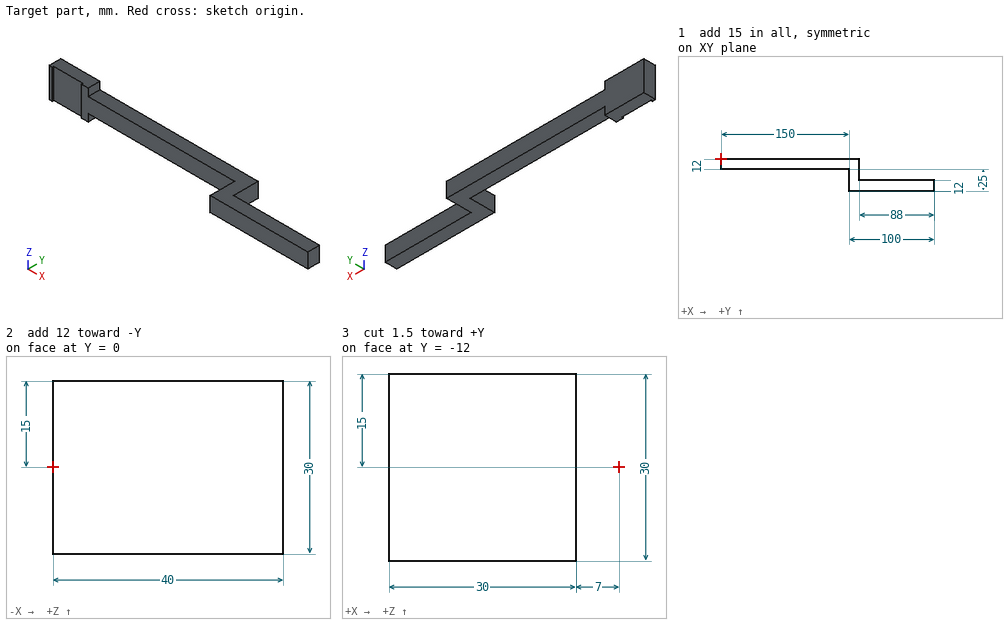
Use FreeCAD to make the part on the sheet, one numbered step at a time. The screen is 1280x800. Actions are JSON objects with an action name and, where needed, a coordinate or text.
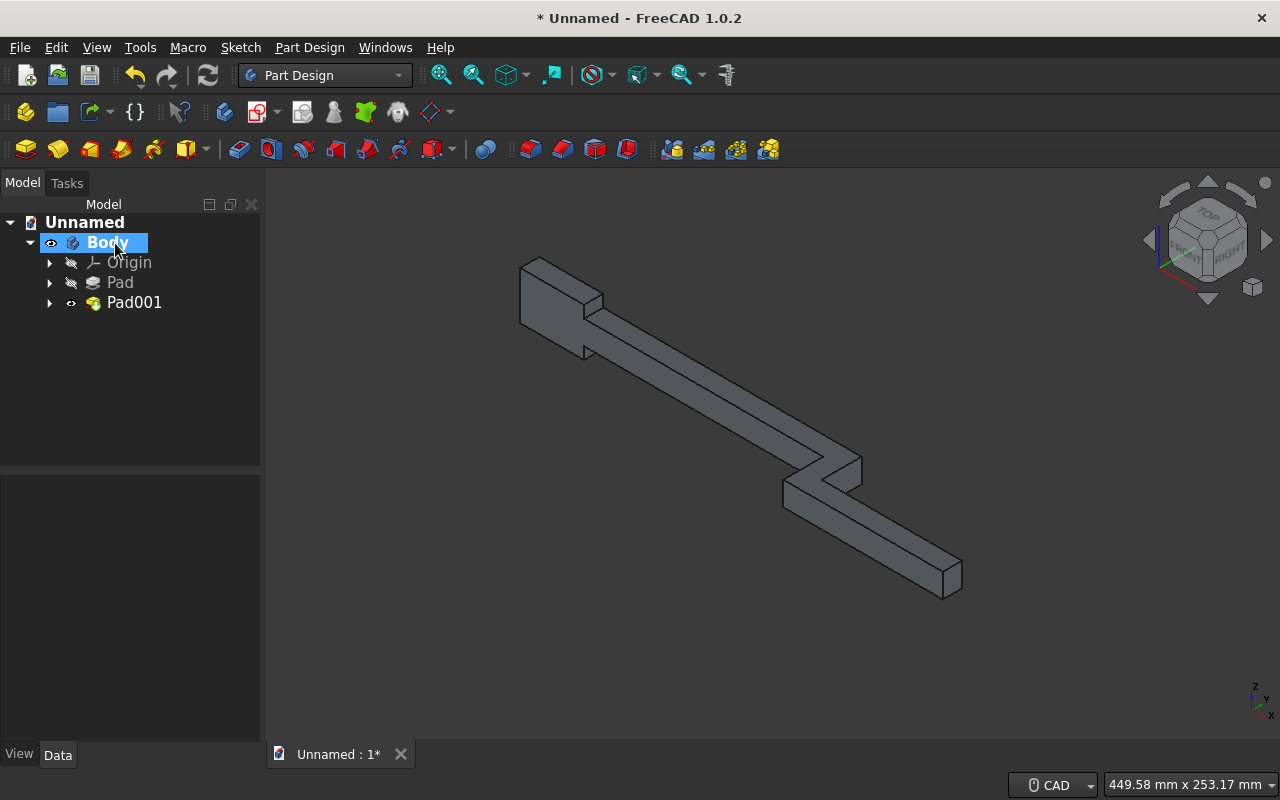
{"action": "left_click", "coordinate": [542, 307]}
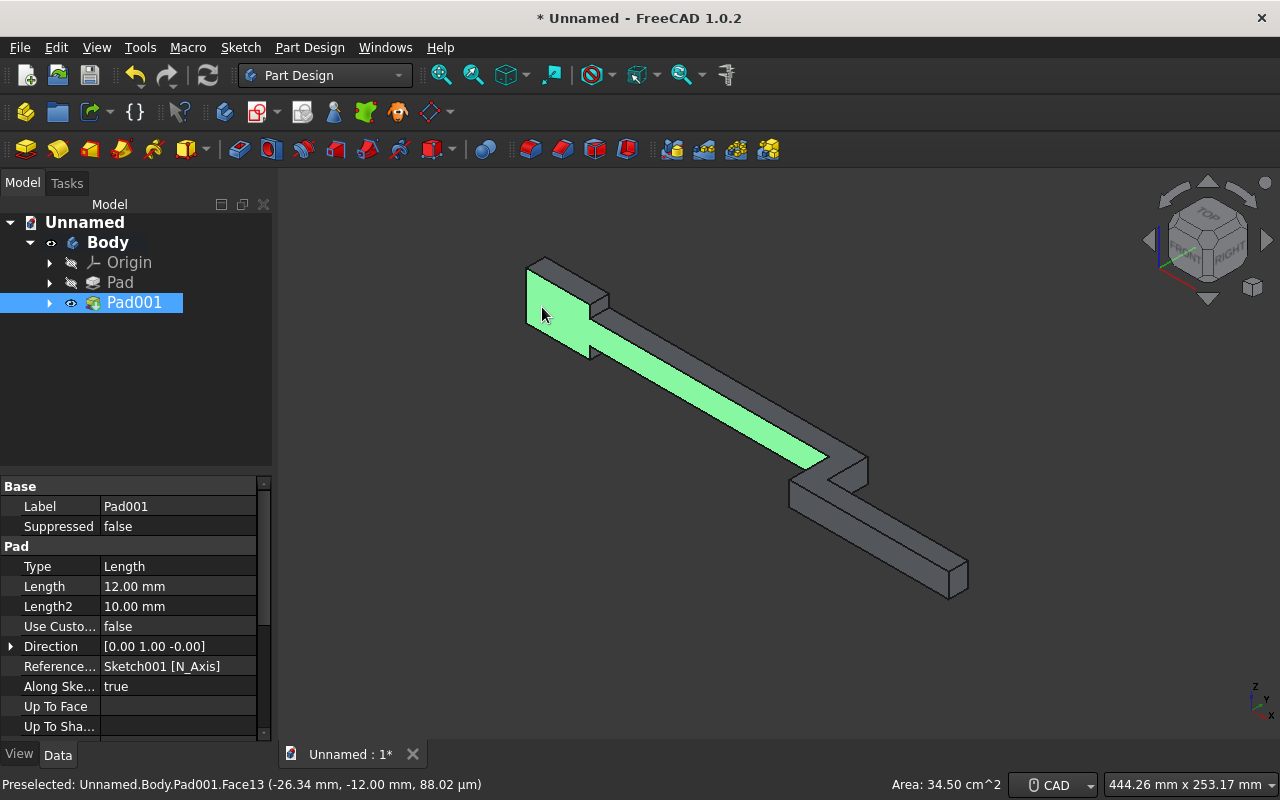
{"action": "left_click", "coordinate": [258, 112]}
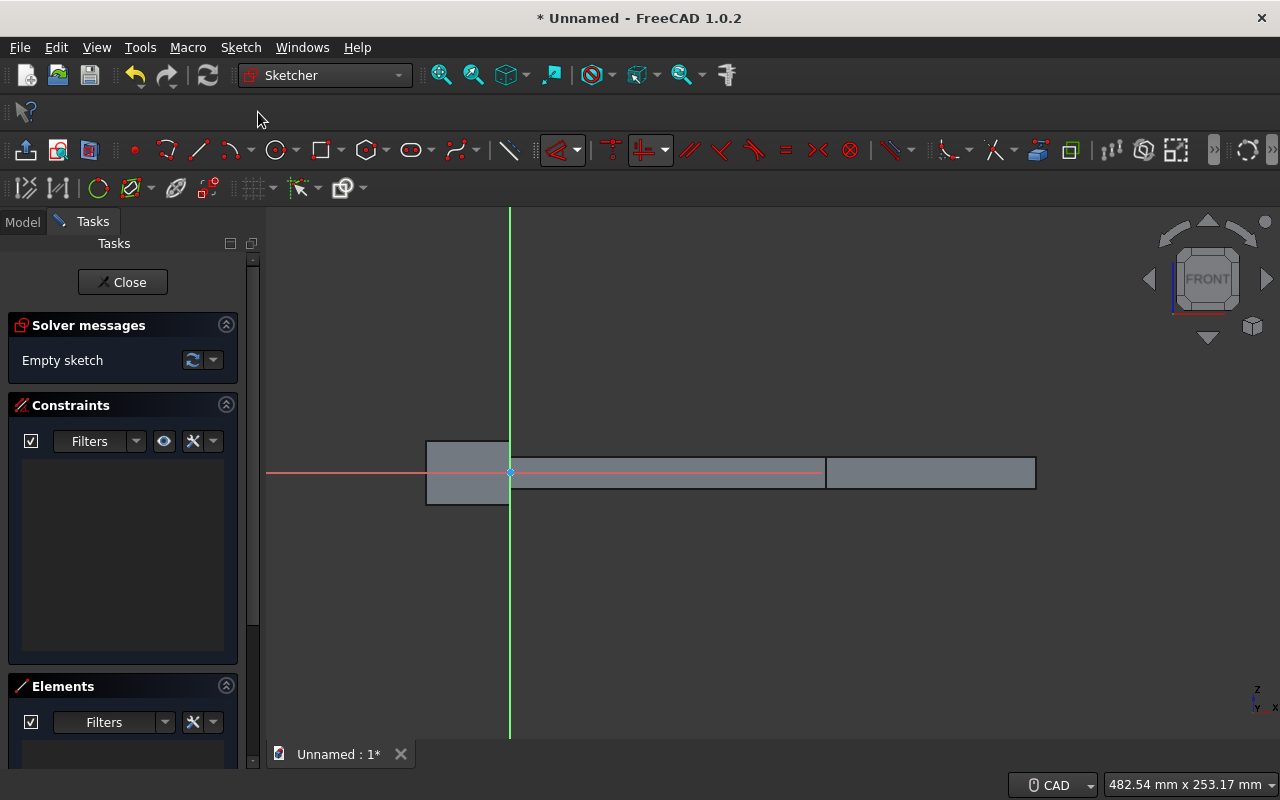
{"action": "left_click", "coordinate": [90, 150]}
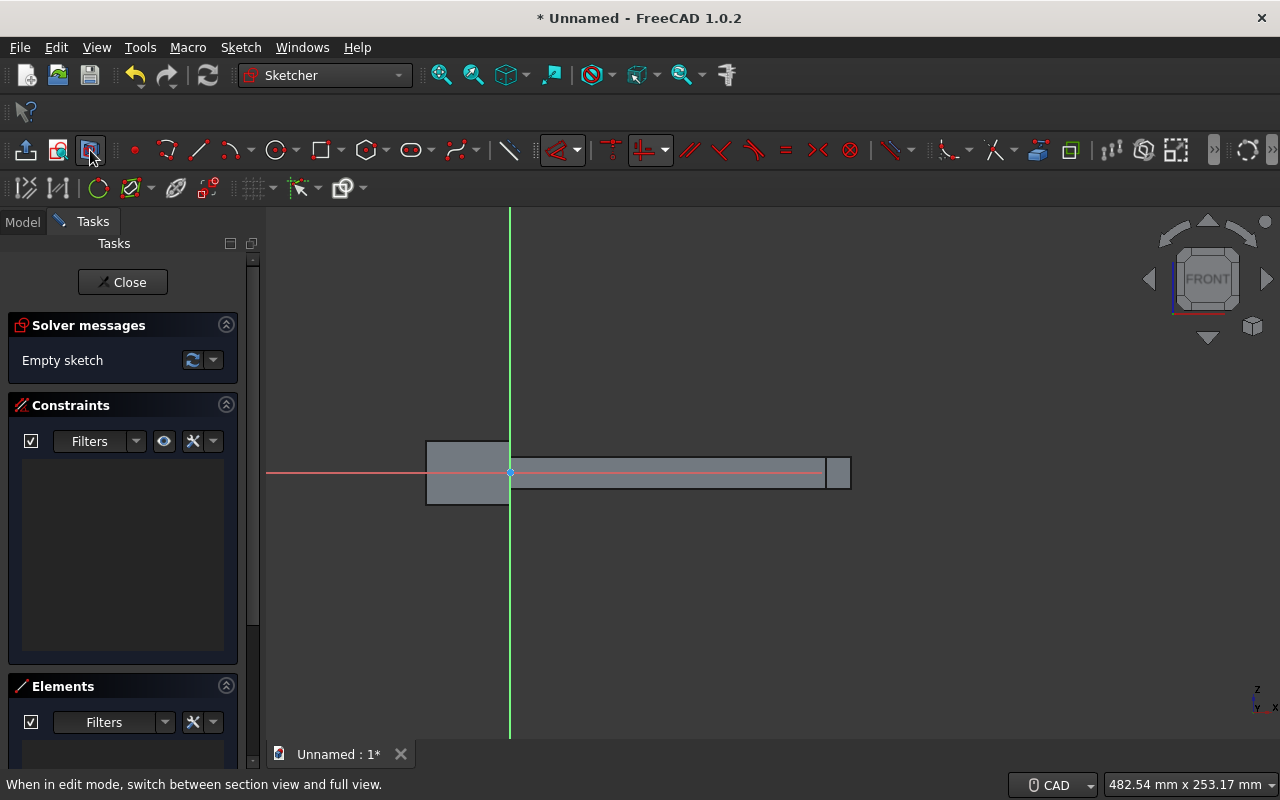
{"action": "scroll", "coordinate": [412, 473], "scroll_direction": "up", "scroll_amount": 8}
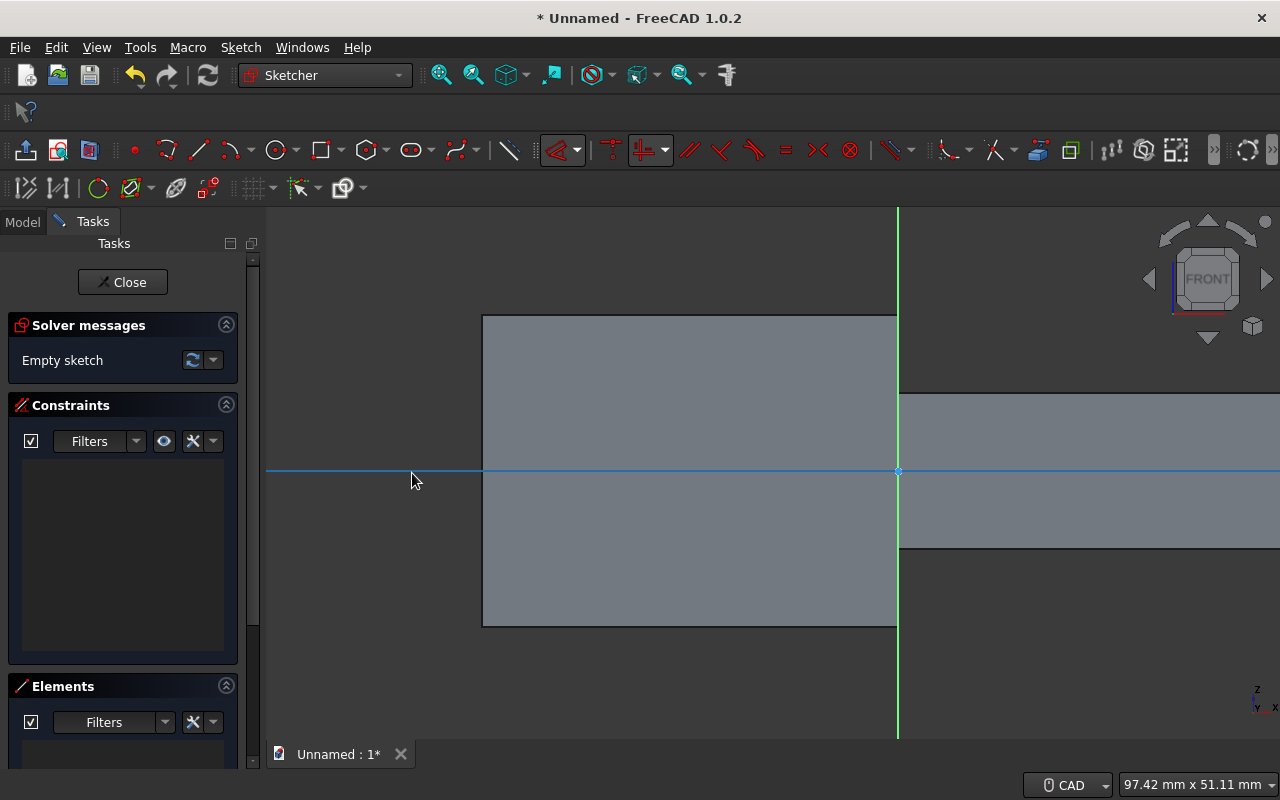
{"action": "left_click", "coordinate": [322, 150]}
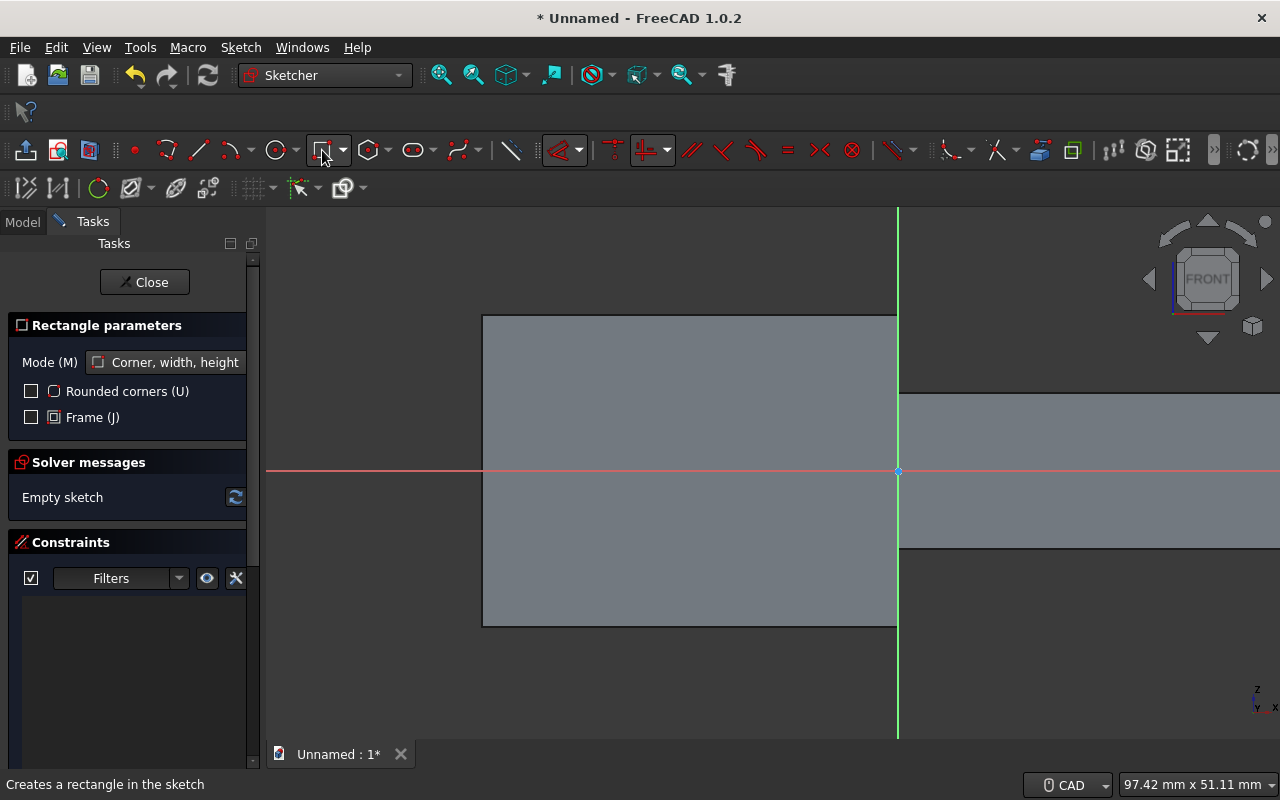
{"action": "left_click", "coordinate": [513, 315]}
{"action": "mouse_move", "coordinate": [826, 627]}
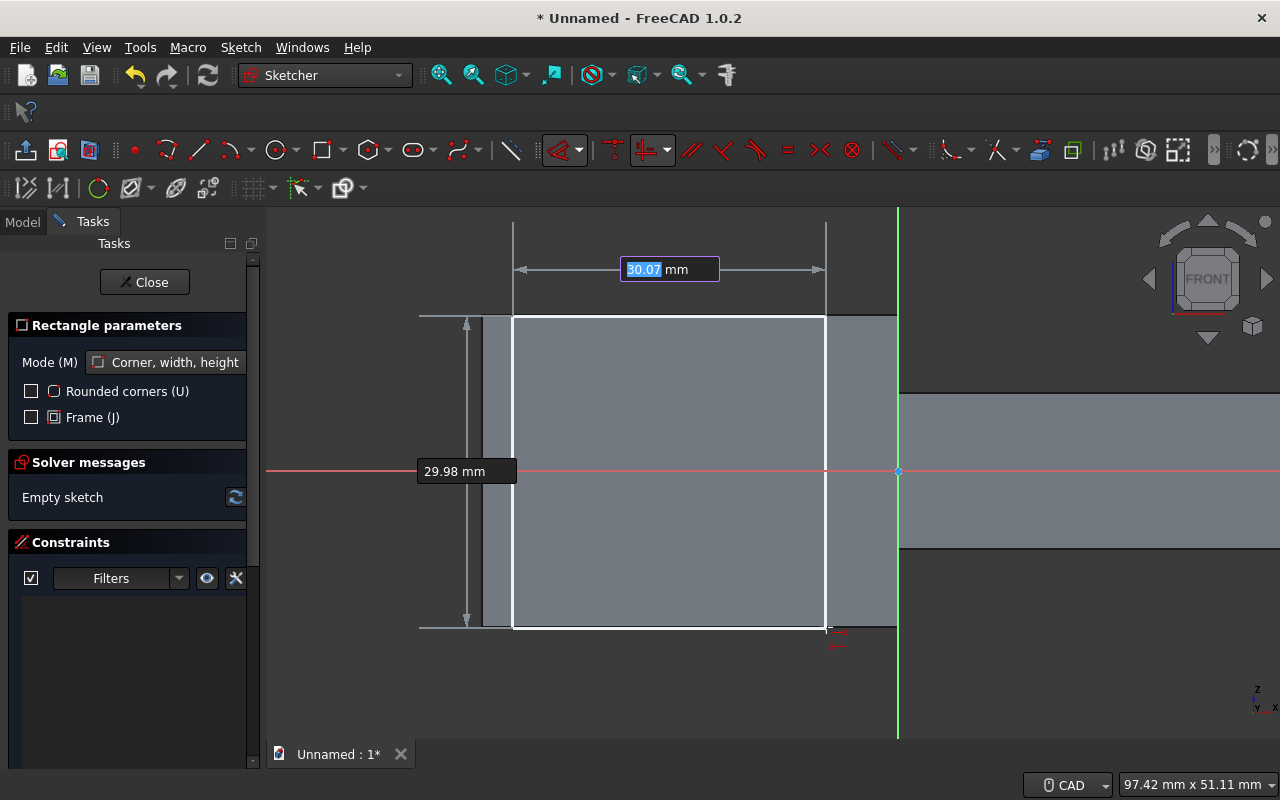
{"action": "type", "text": "30"}
{"action": "key", "text": "Tab"}
{"action": "type", "text": "30"}
{"action": "key", "text": "Return"}
{"action": "key", "text": "Escape"}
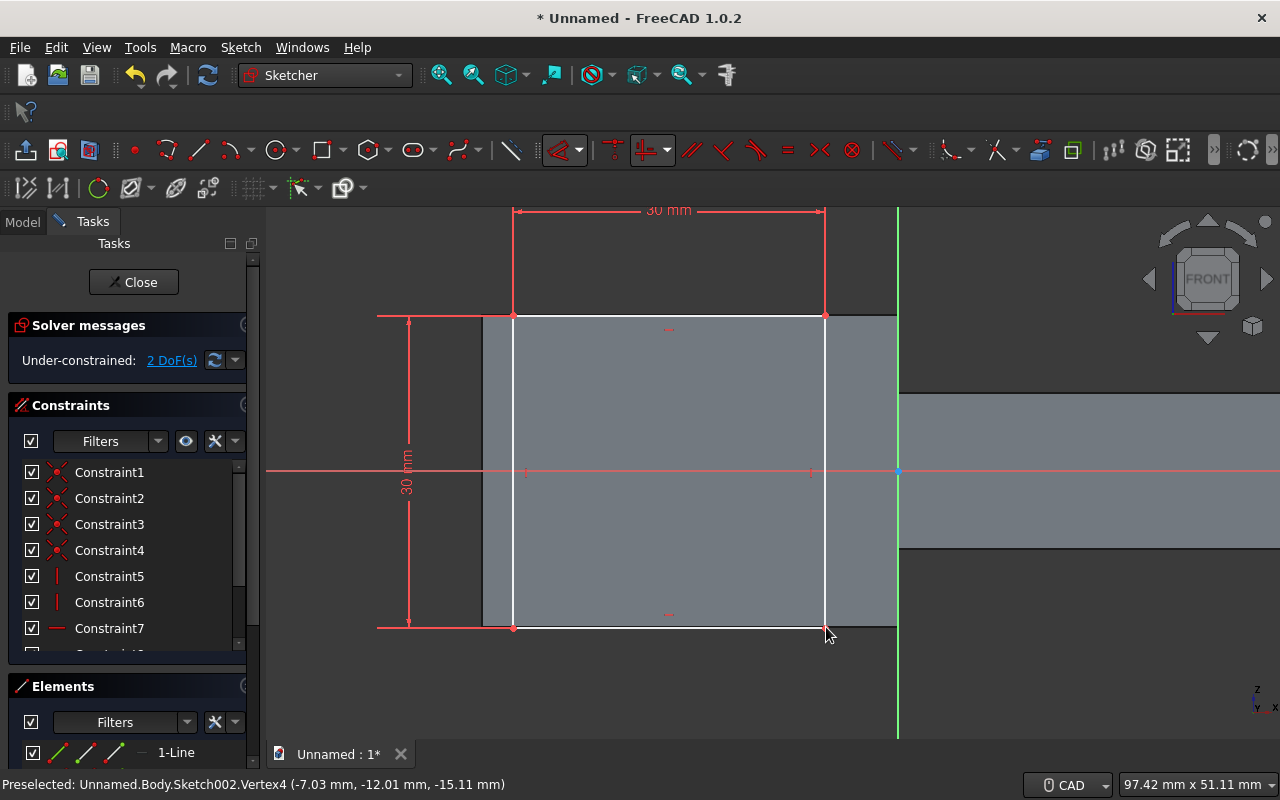
{"action": "left_click", "coordinate": [825, 628]}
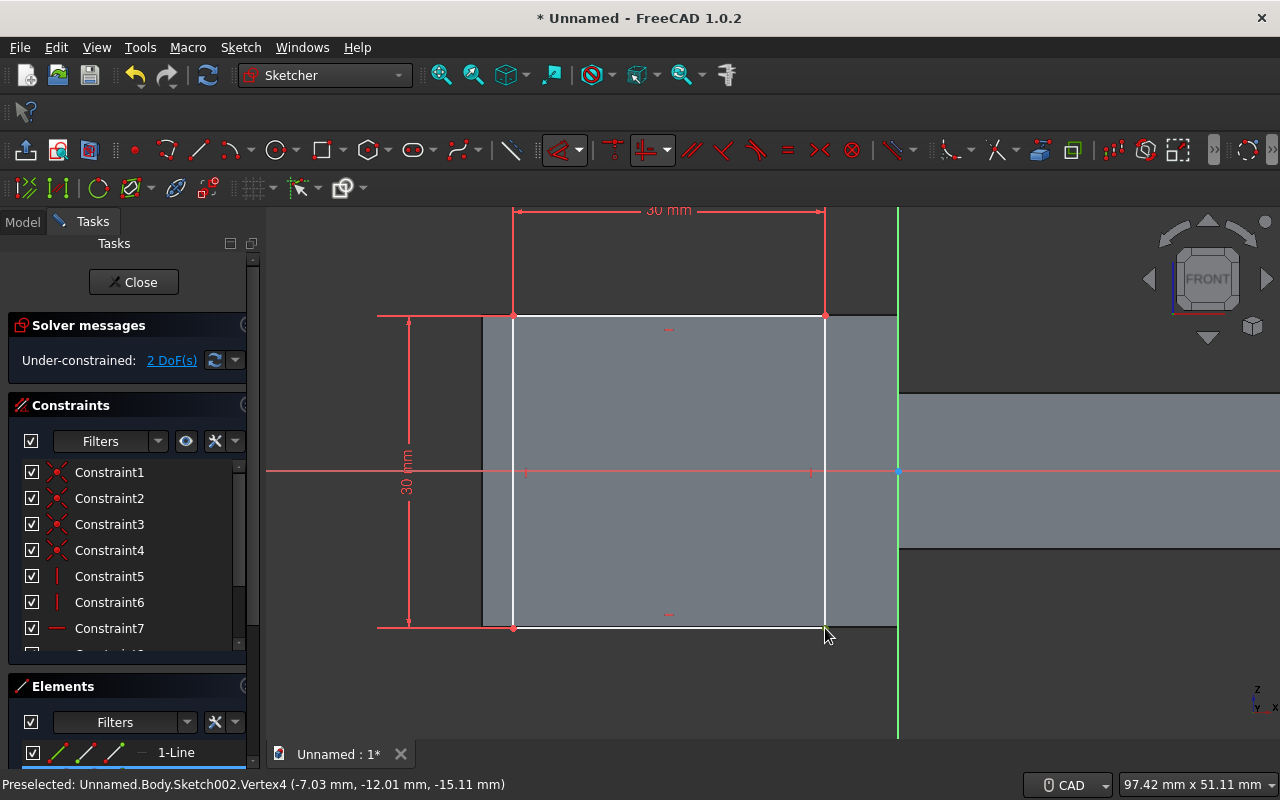
{"action": "key", "text": "l"}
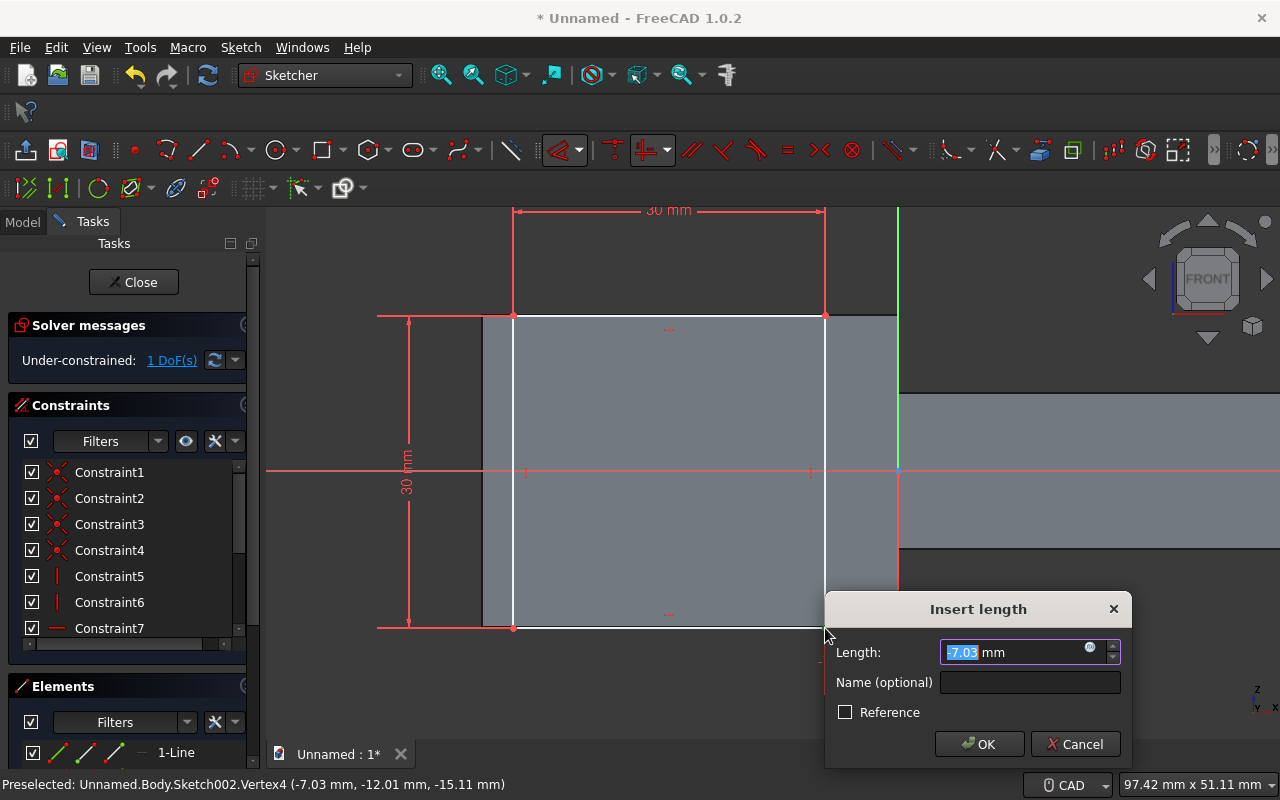
{"action": "type", "text": "-7"}
{"action": "key", "text": "Return"}